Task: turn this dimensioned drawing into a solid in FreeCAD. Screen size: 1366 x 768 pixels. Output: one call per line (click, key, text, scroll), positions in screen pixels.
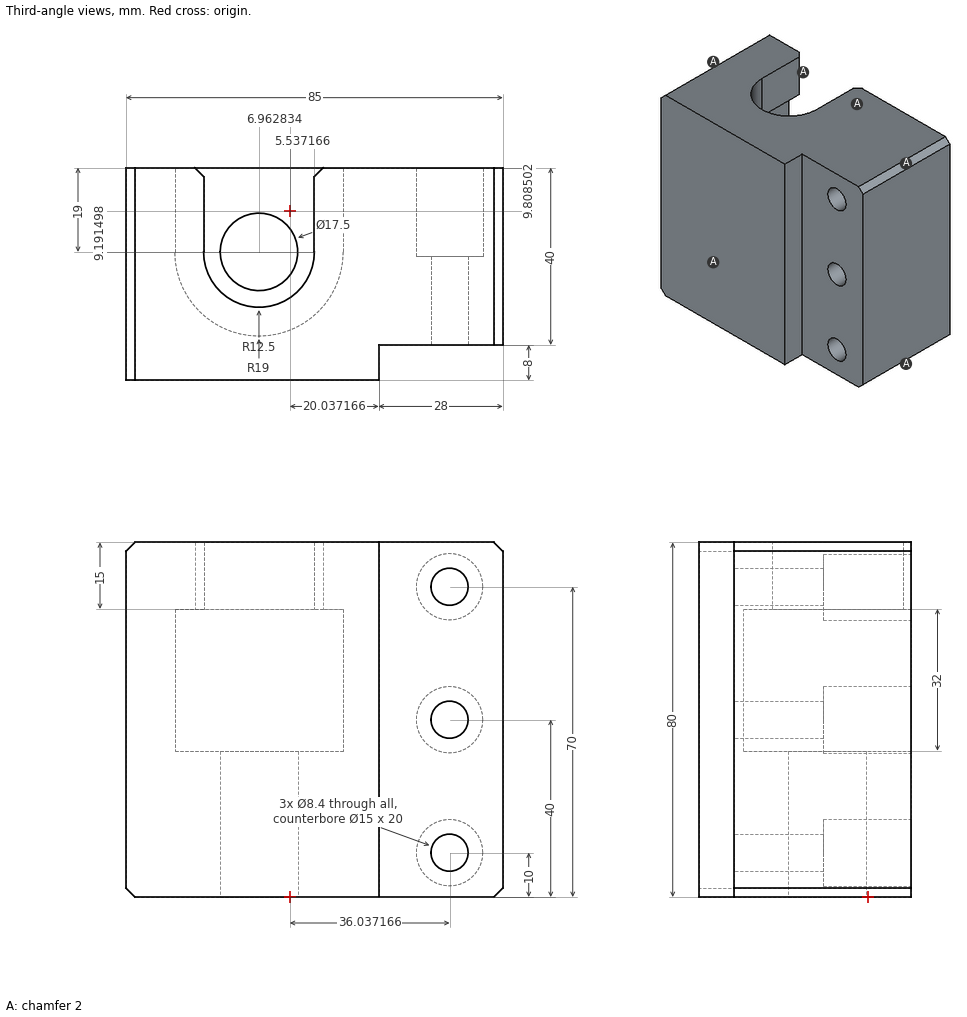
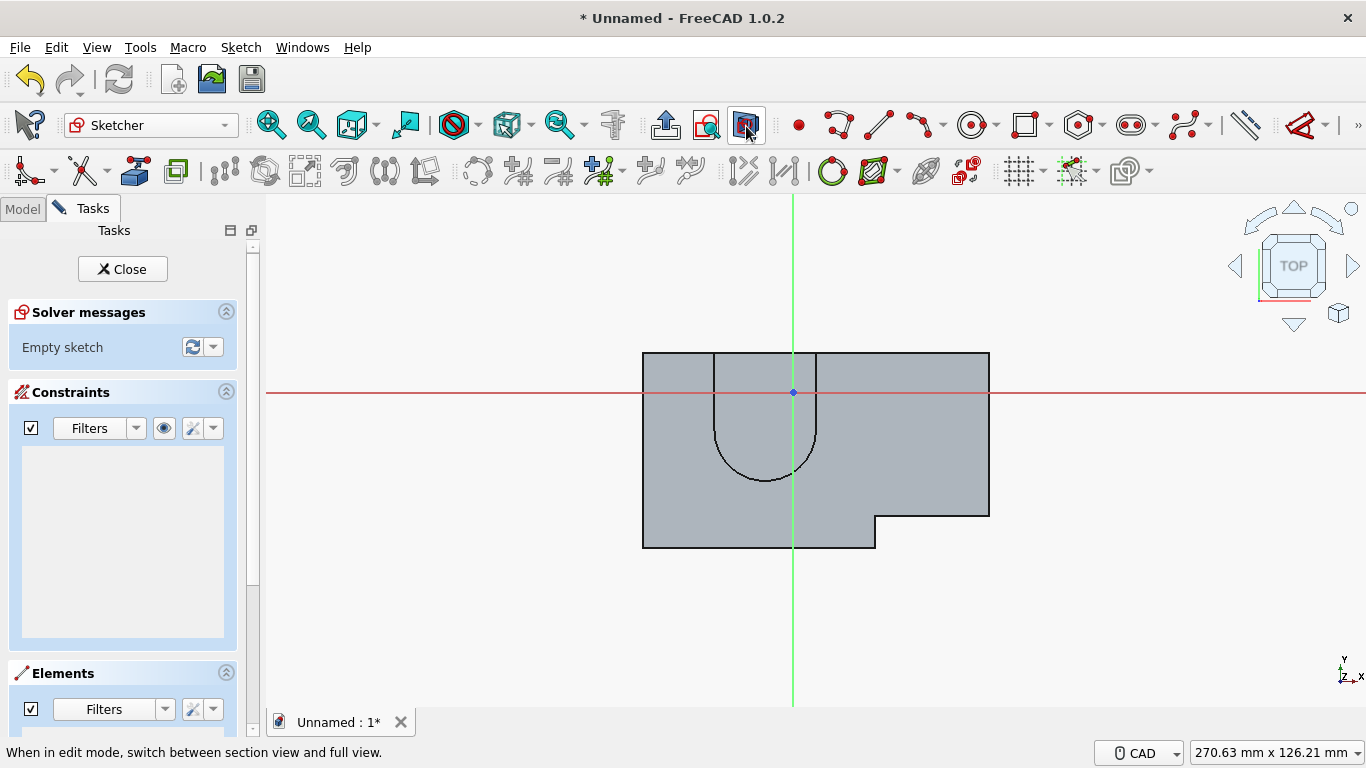
scroll(780, 414, up, 4)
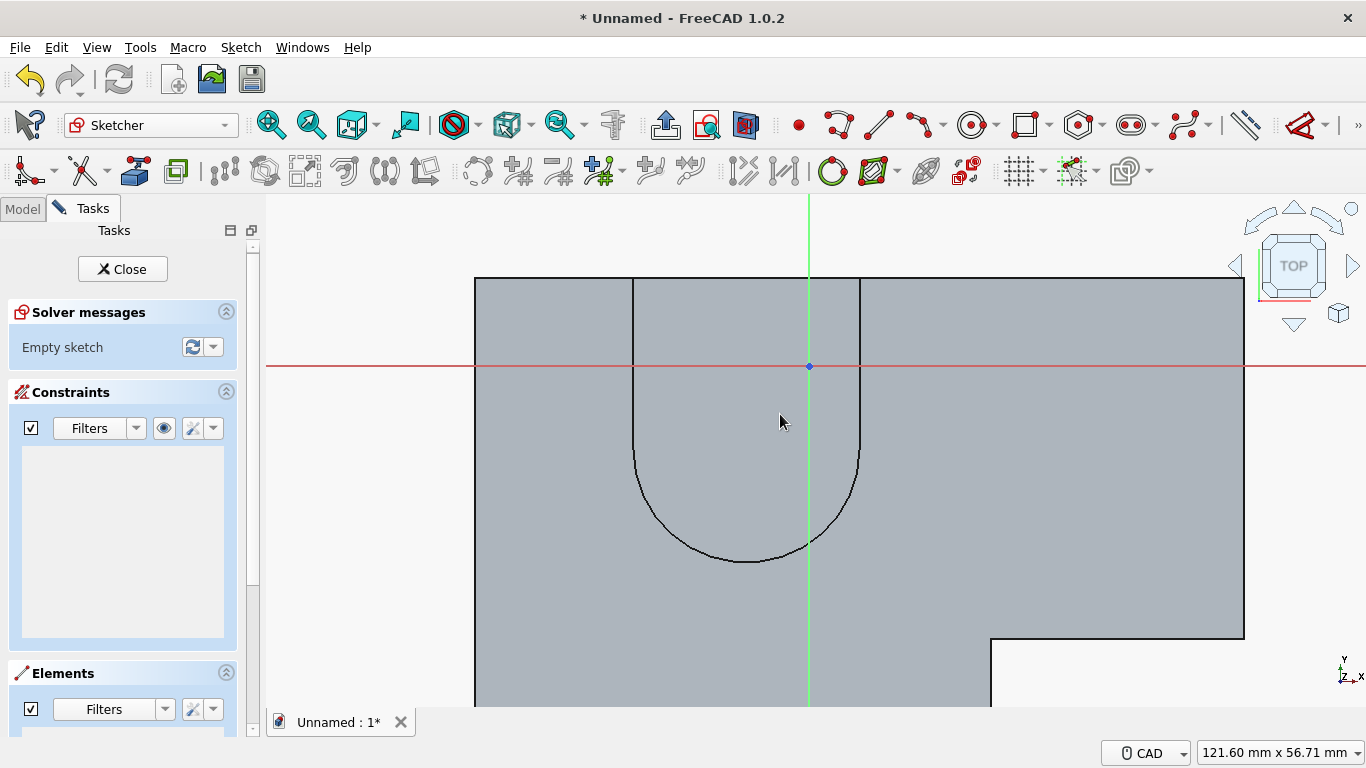
click(840, 126)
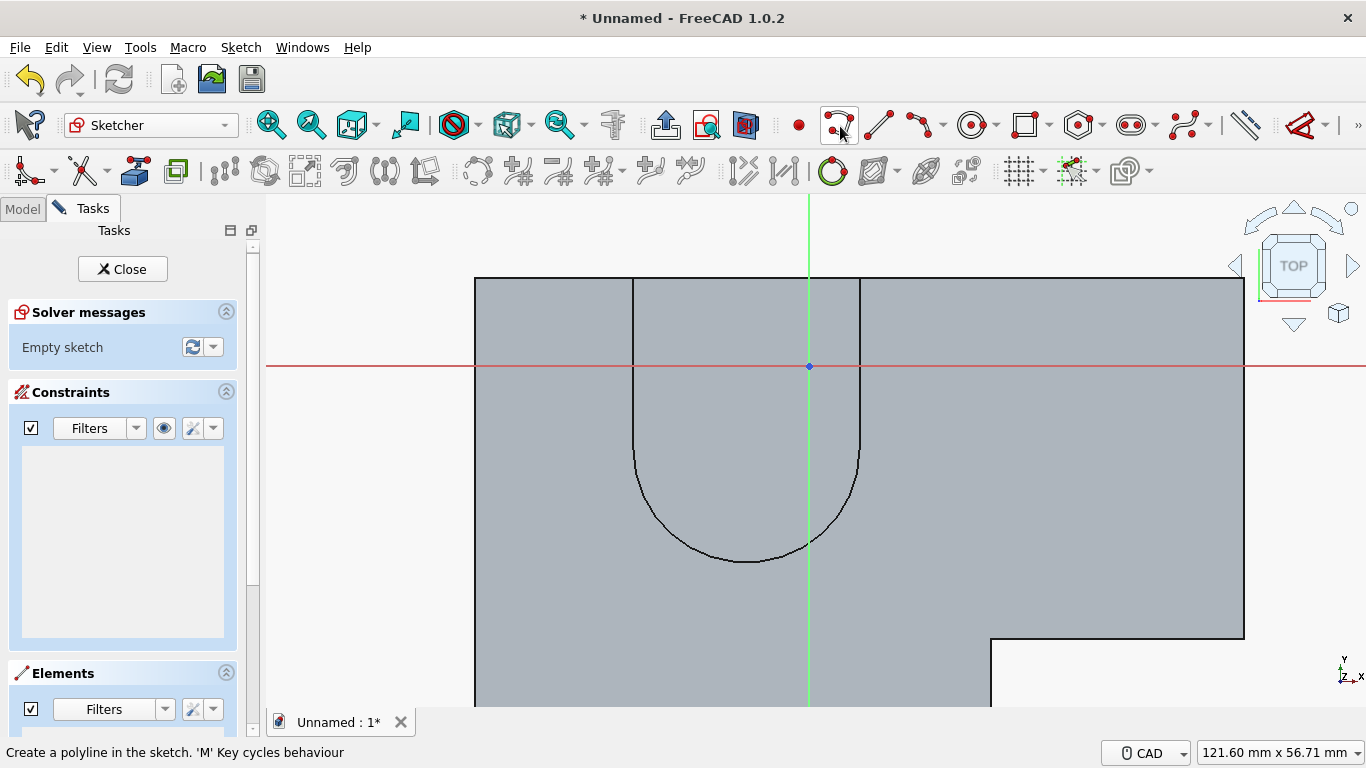
click(918, 449)
click(918, 278)
click(575, 278)
click(575, 449)
right_click(575, 449)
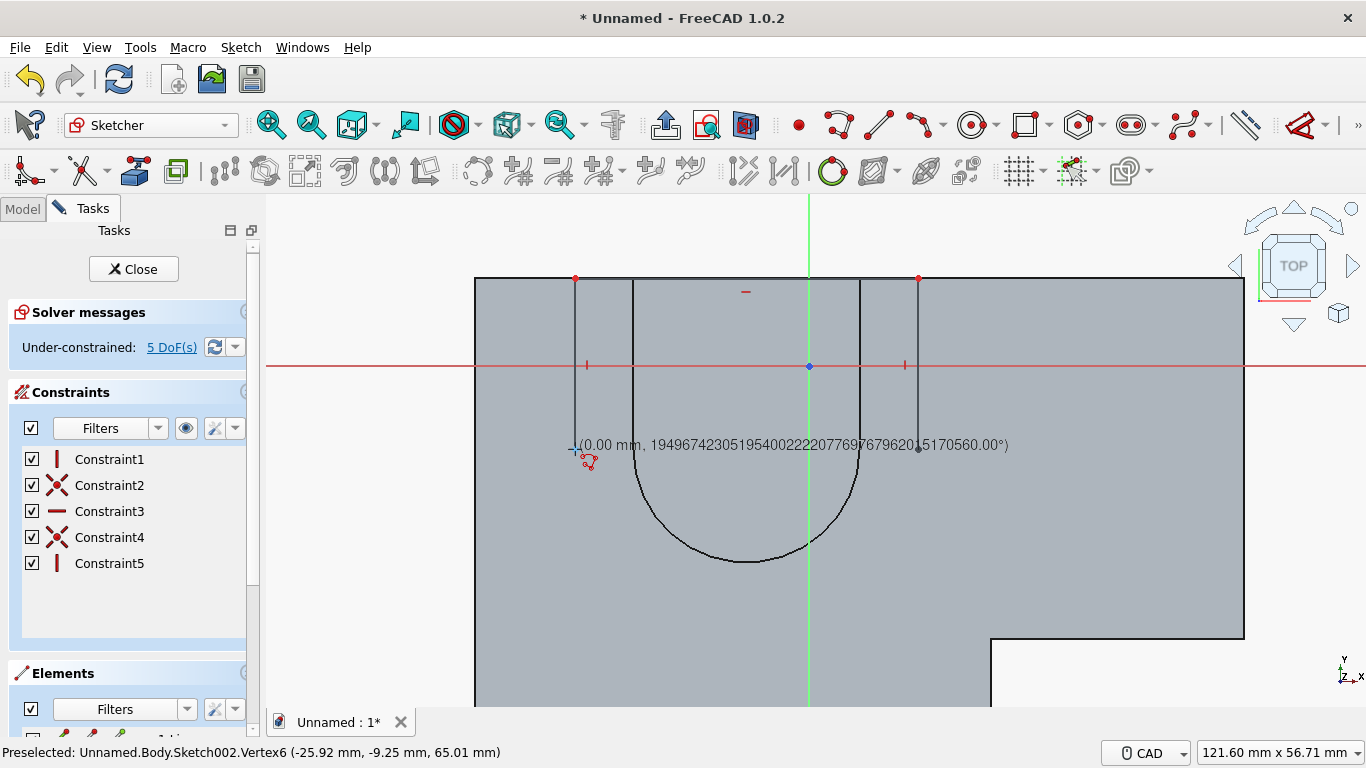
click(920, 126)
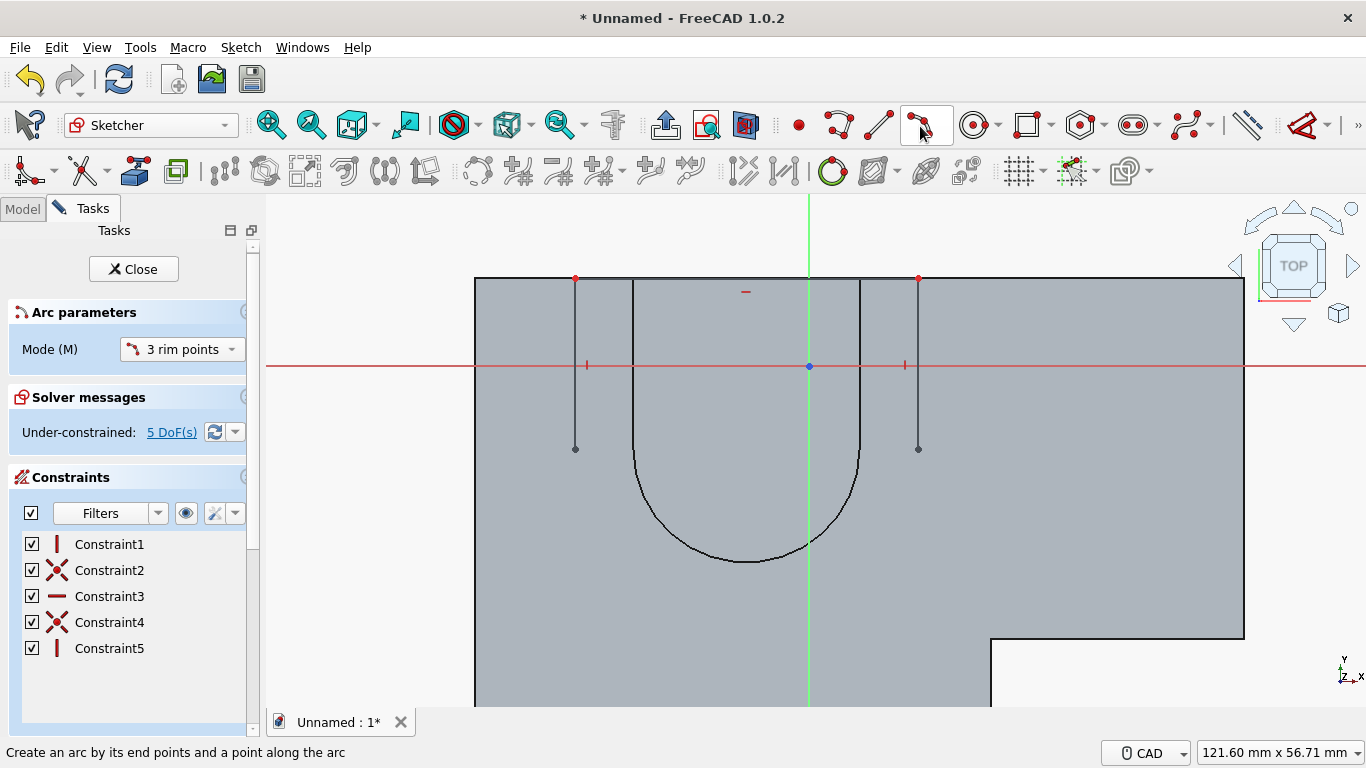
click(575, 450)
click(918, 450)
click(746, 621)
key(Escape)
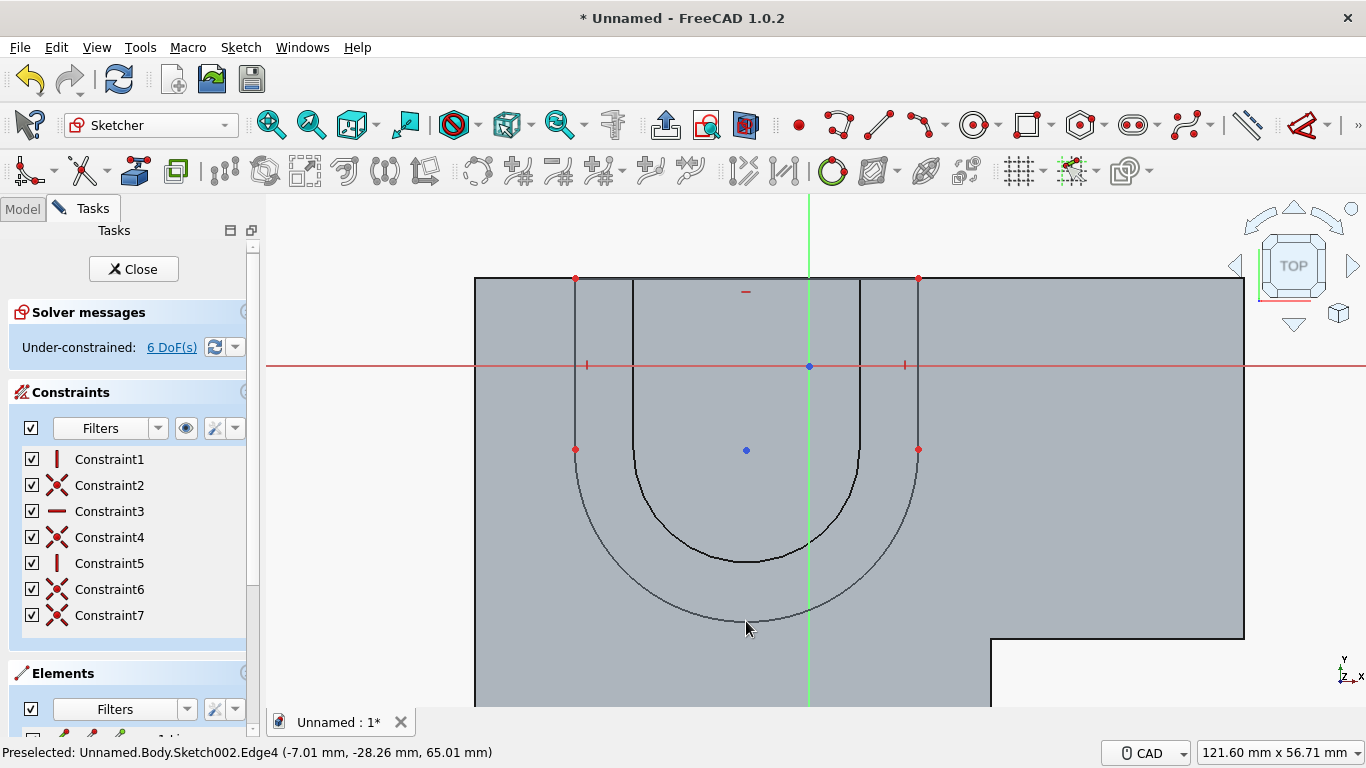
click(918, 399)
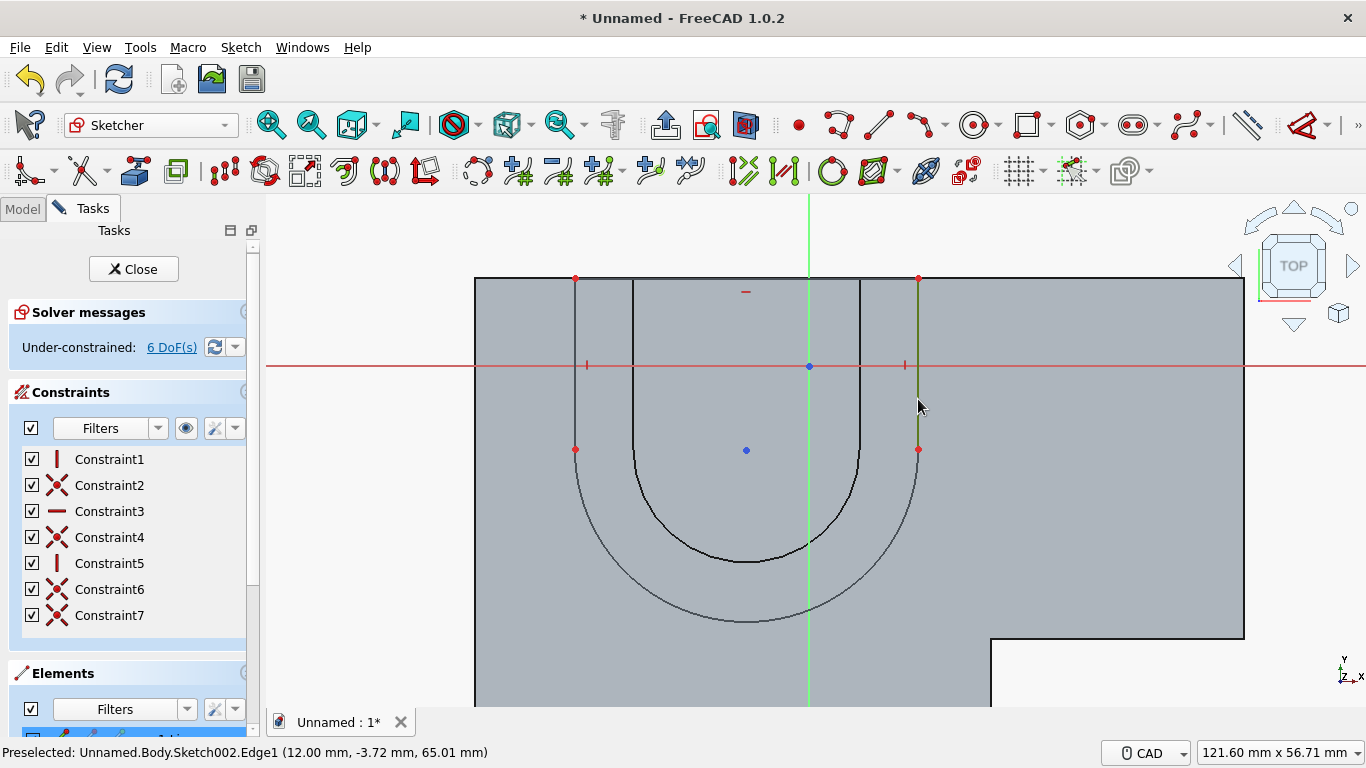
click(646, 589)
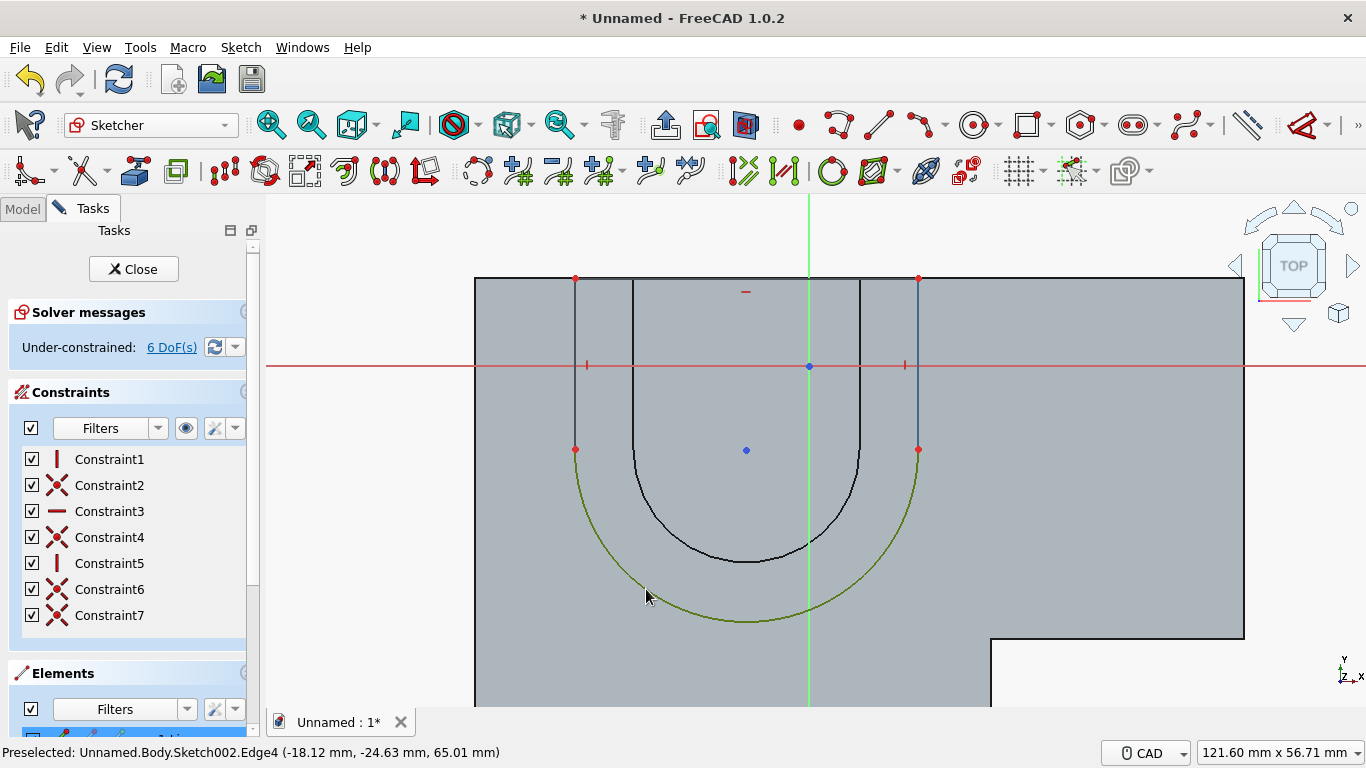
key(t)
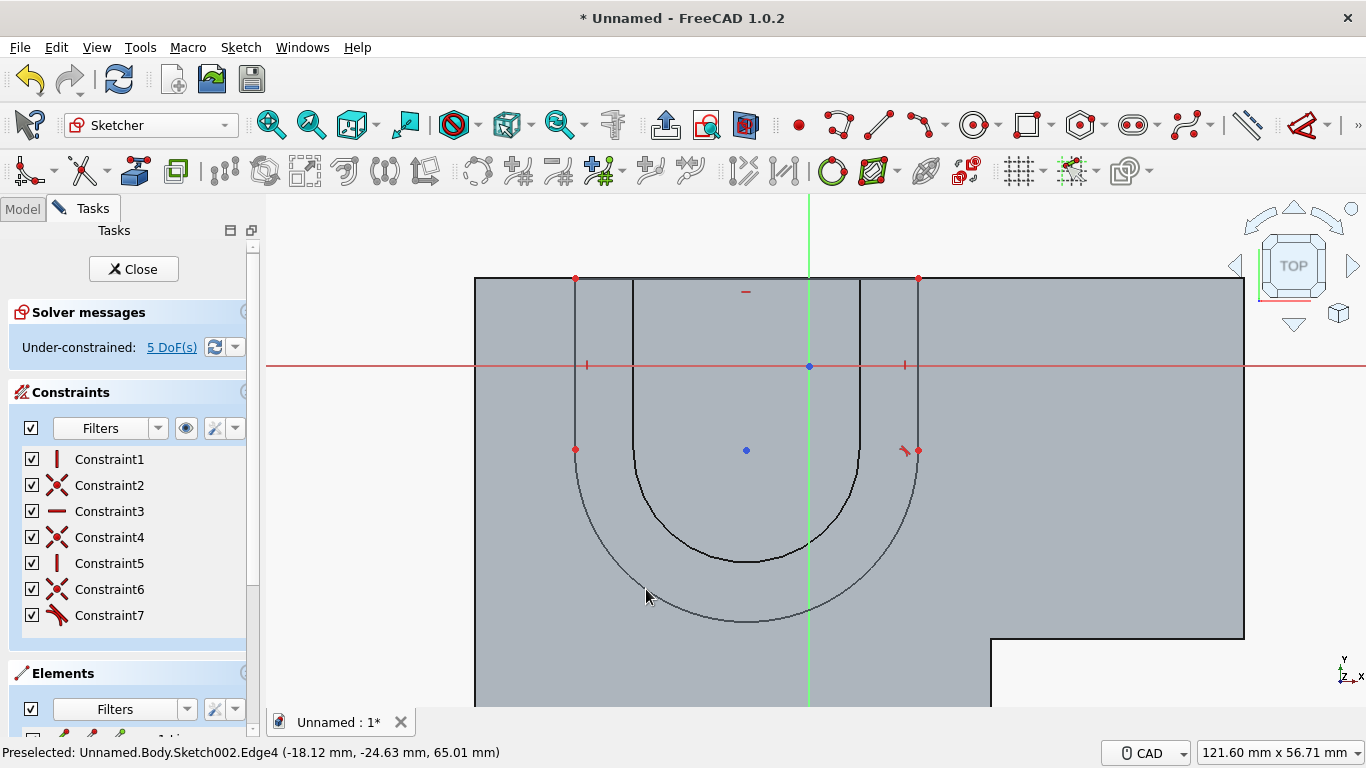
click(575, 330)